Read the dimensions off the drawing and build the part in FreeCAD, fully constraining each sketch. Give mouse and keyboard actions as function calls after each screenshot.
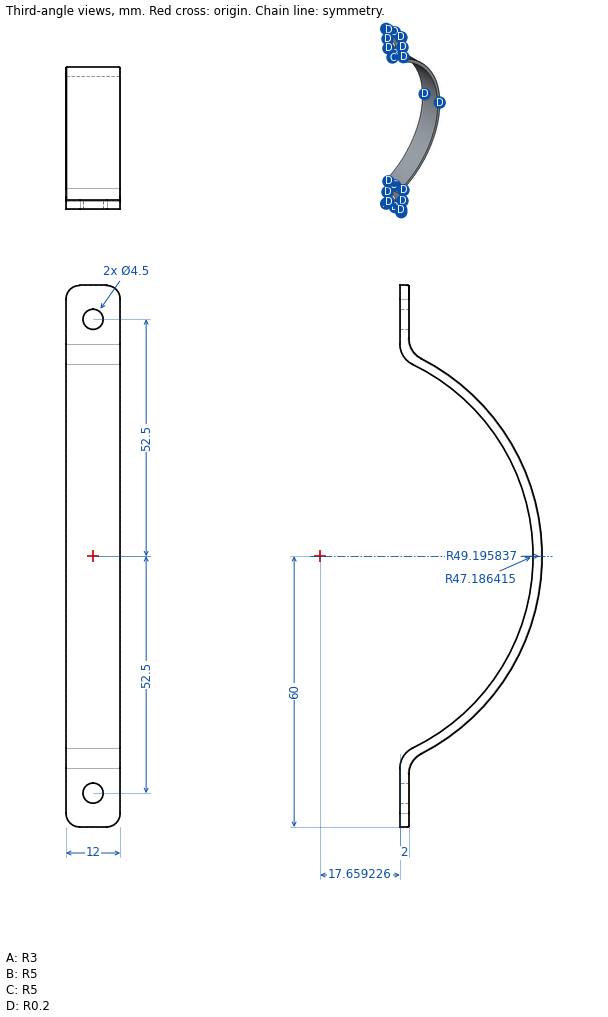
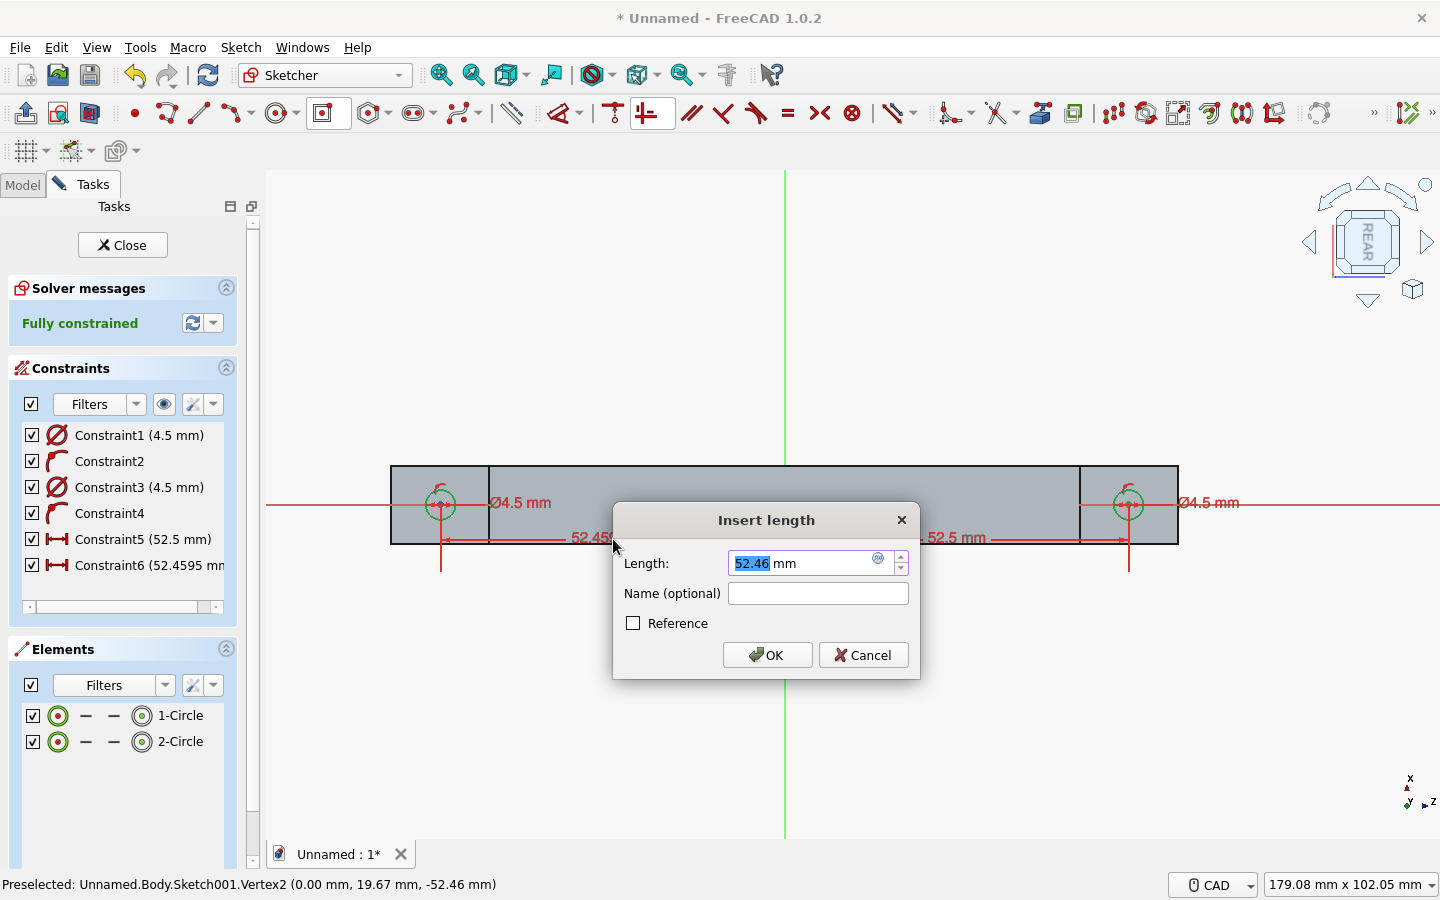
text(52.5)
key(Return)
key(Escape)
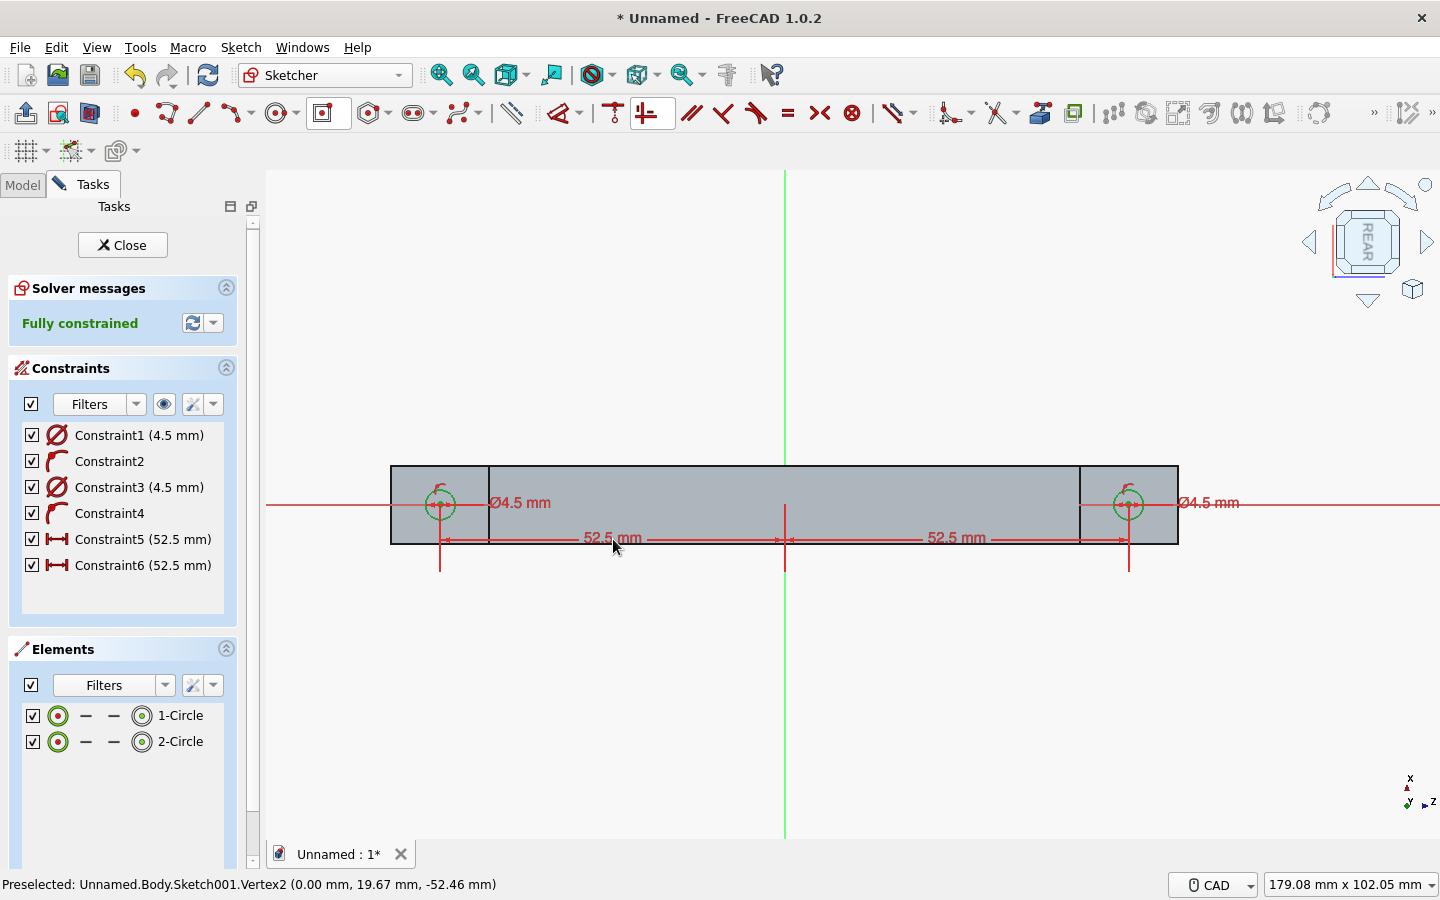
click(123, 245)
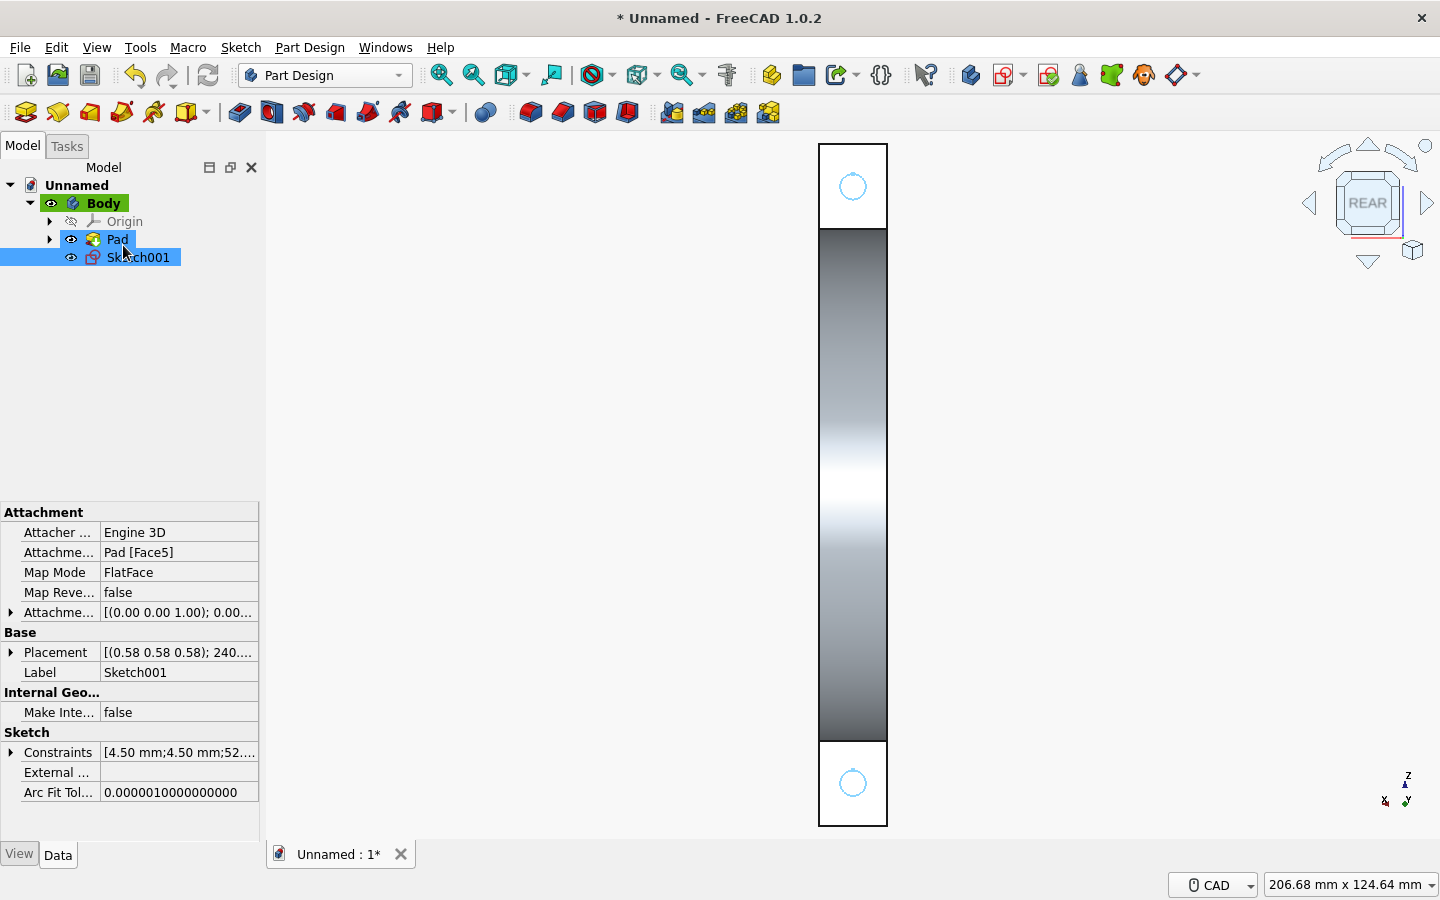
click(240, 112)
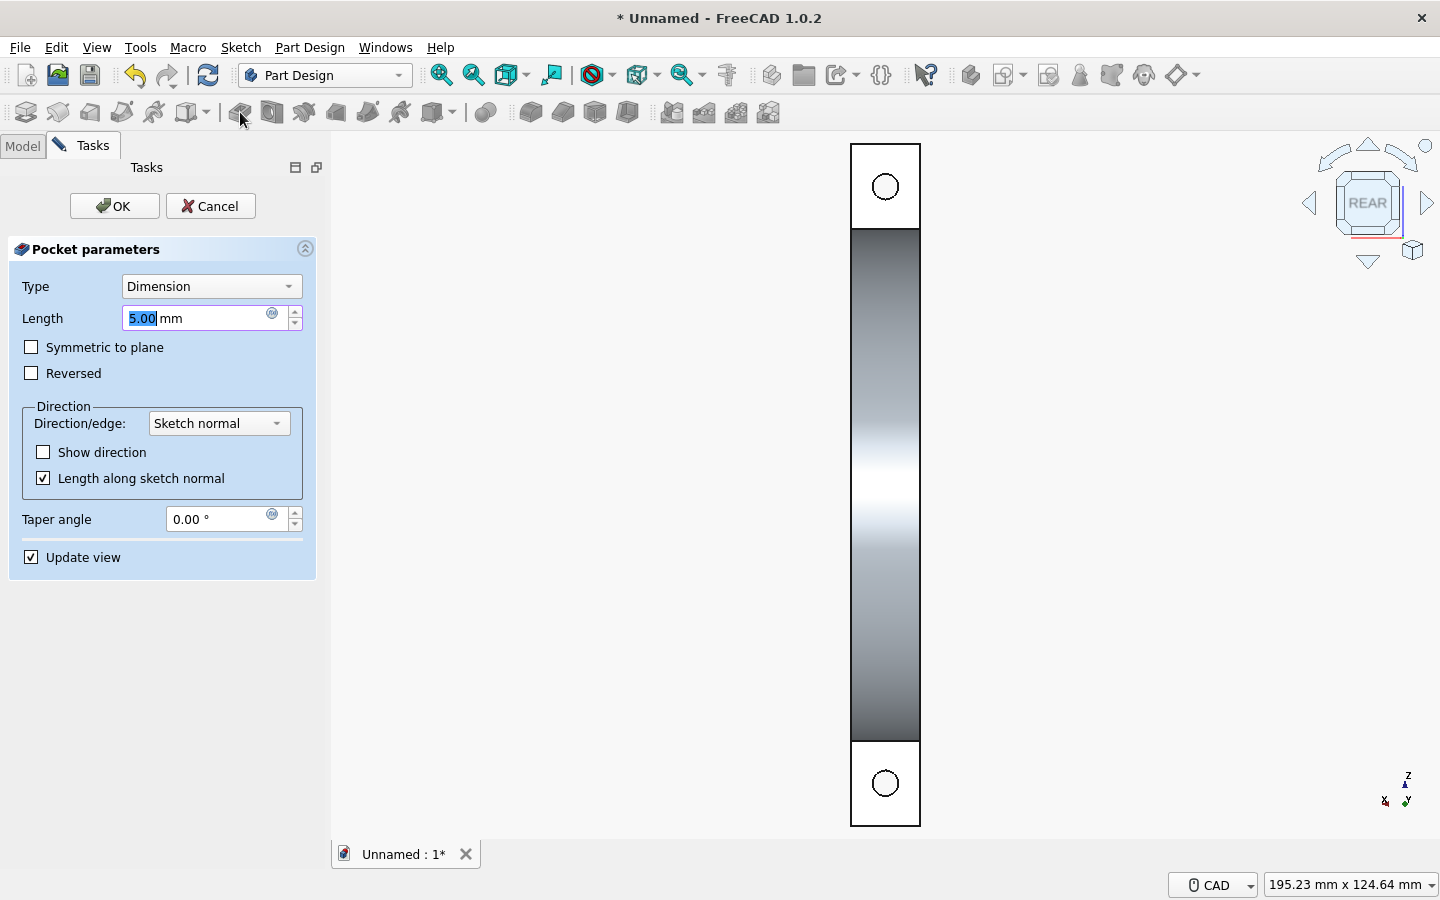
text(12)
key(Tab)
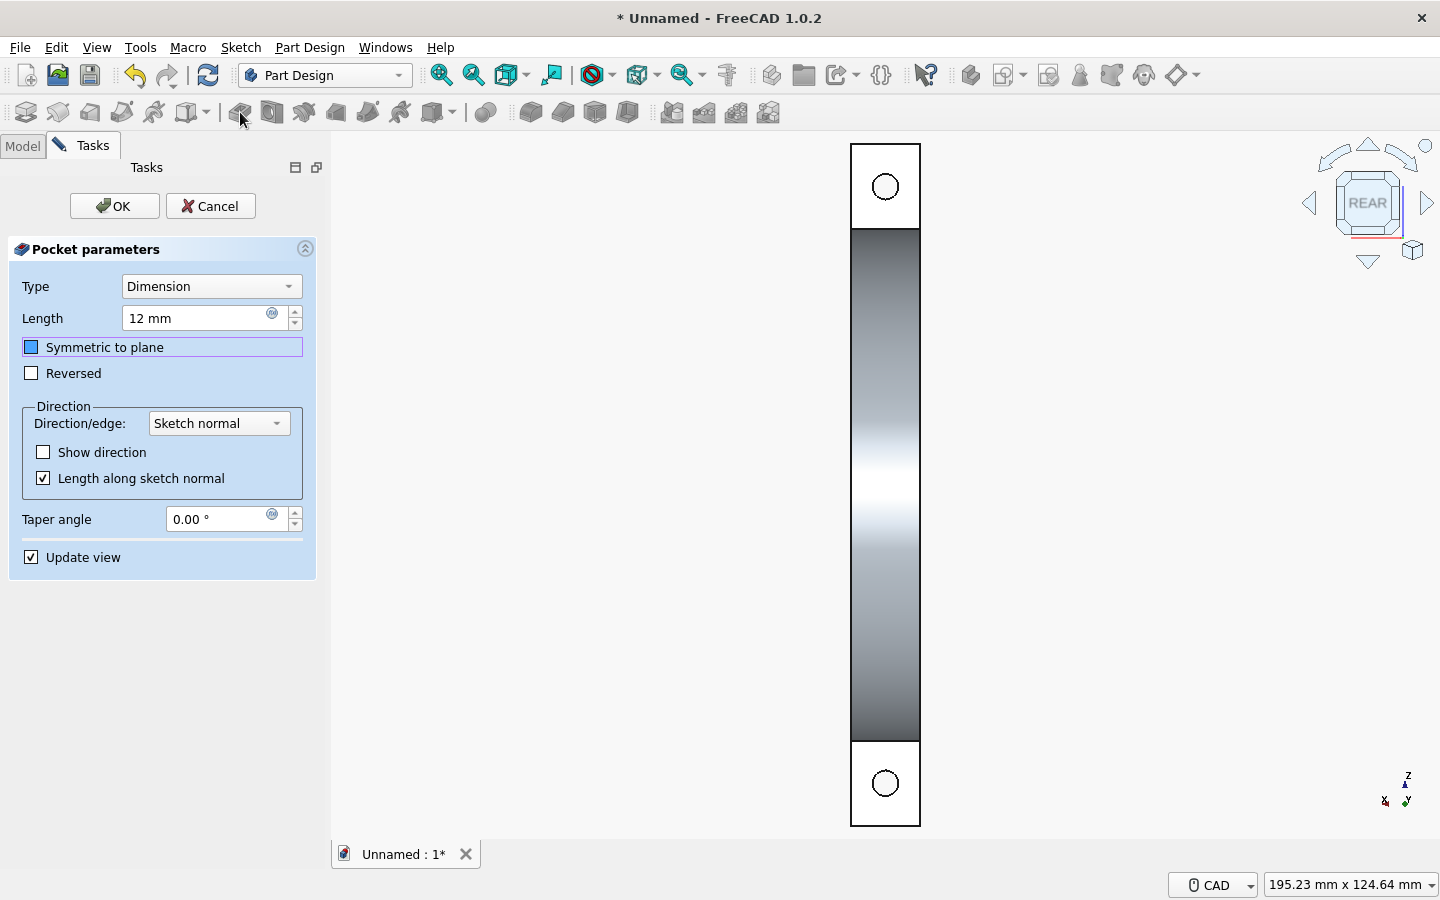
click(115, 206)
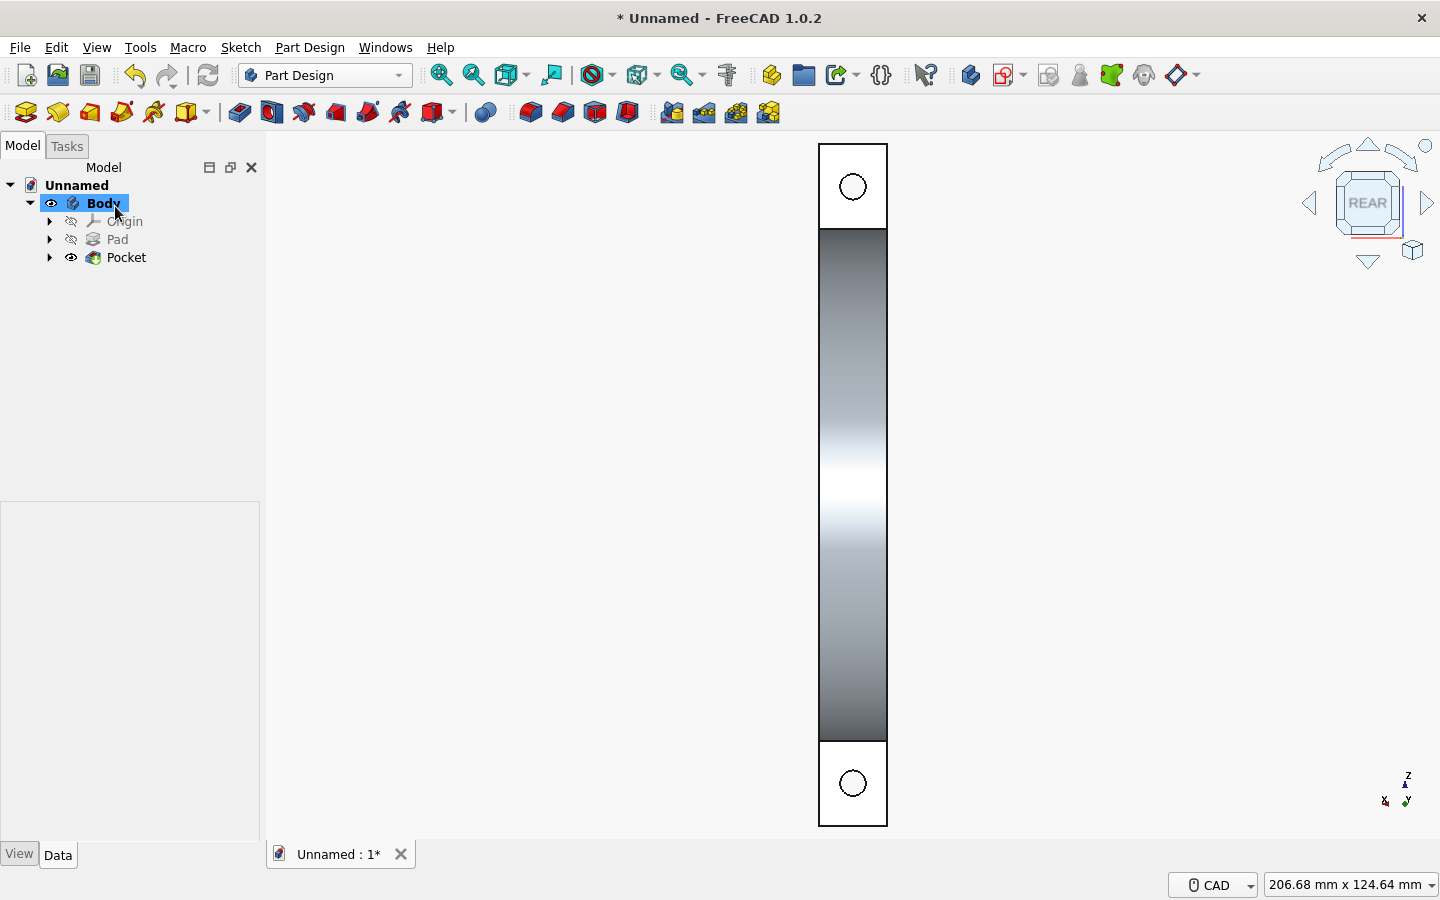
key(0)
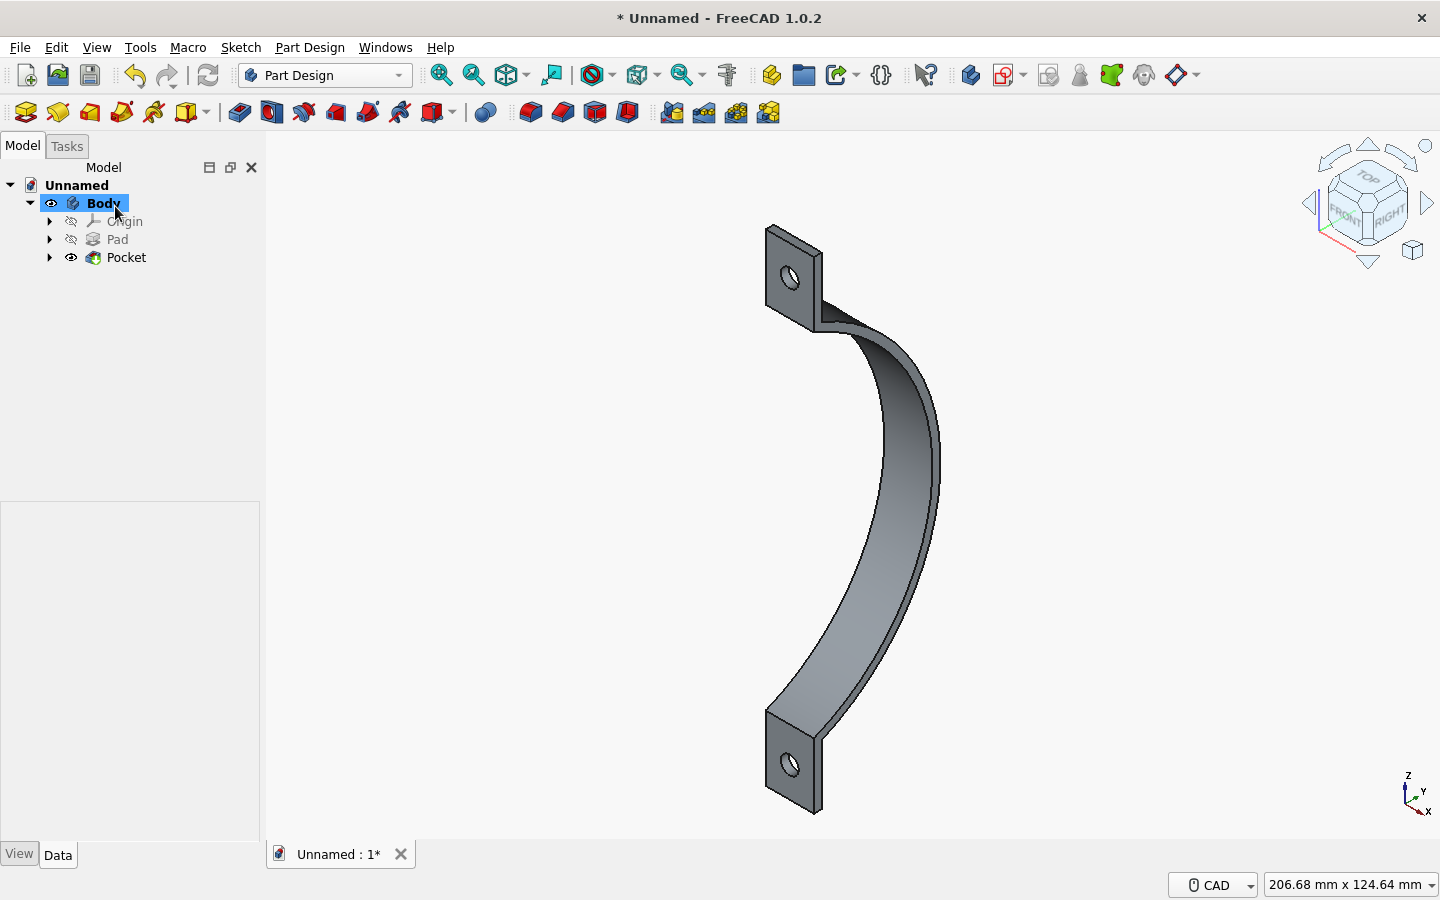
scroll(818, 810, up, 7)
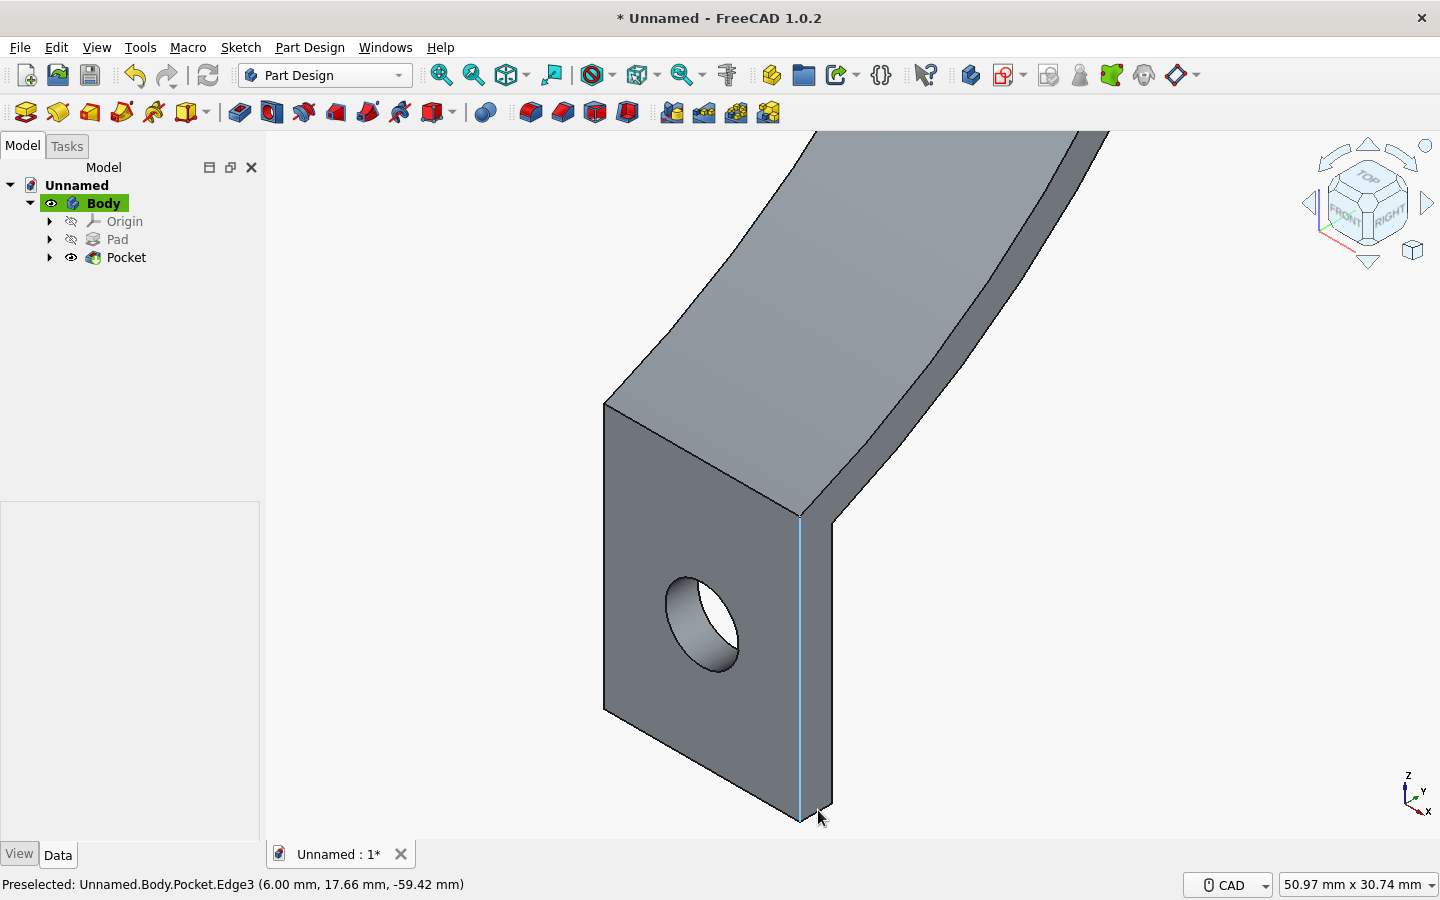
click(442, 76)